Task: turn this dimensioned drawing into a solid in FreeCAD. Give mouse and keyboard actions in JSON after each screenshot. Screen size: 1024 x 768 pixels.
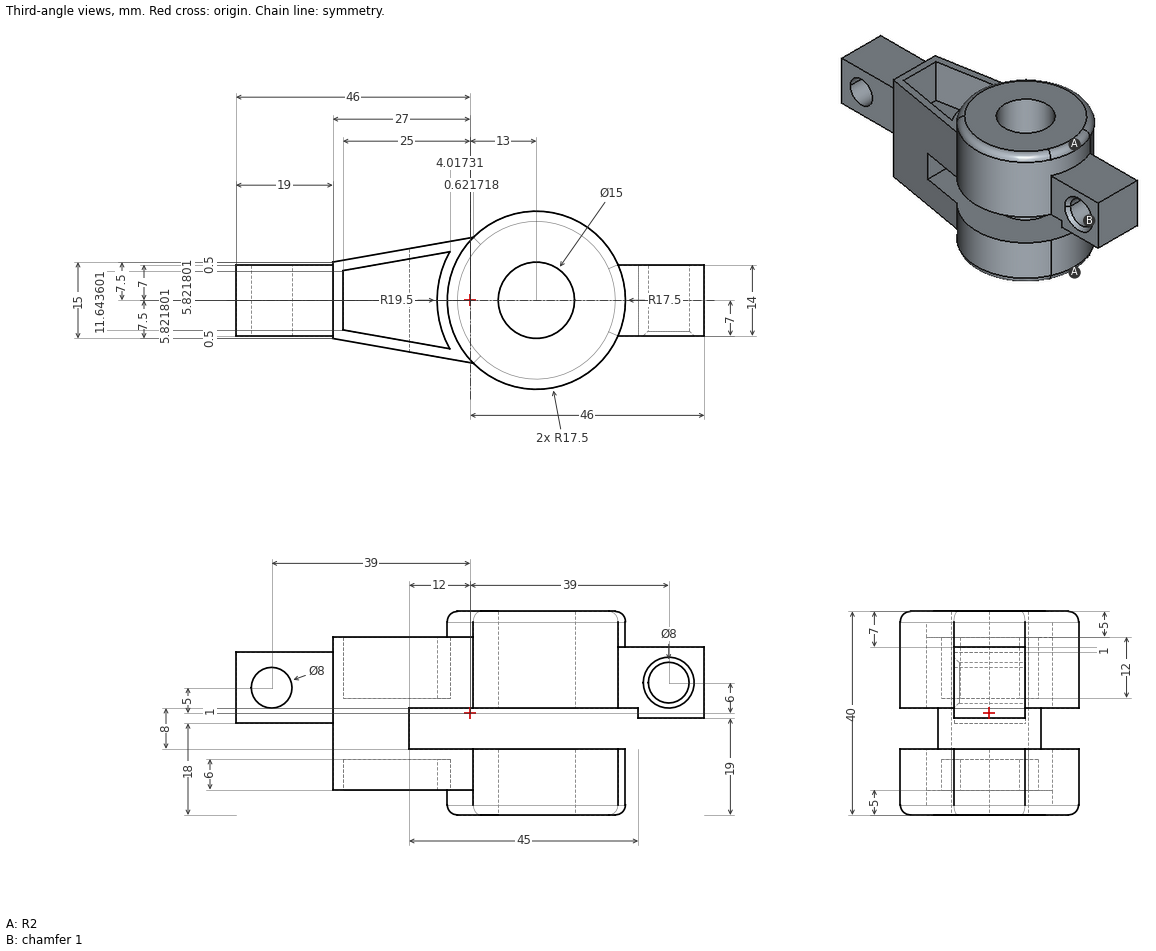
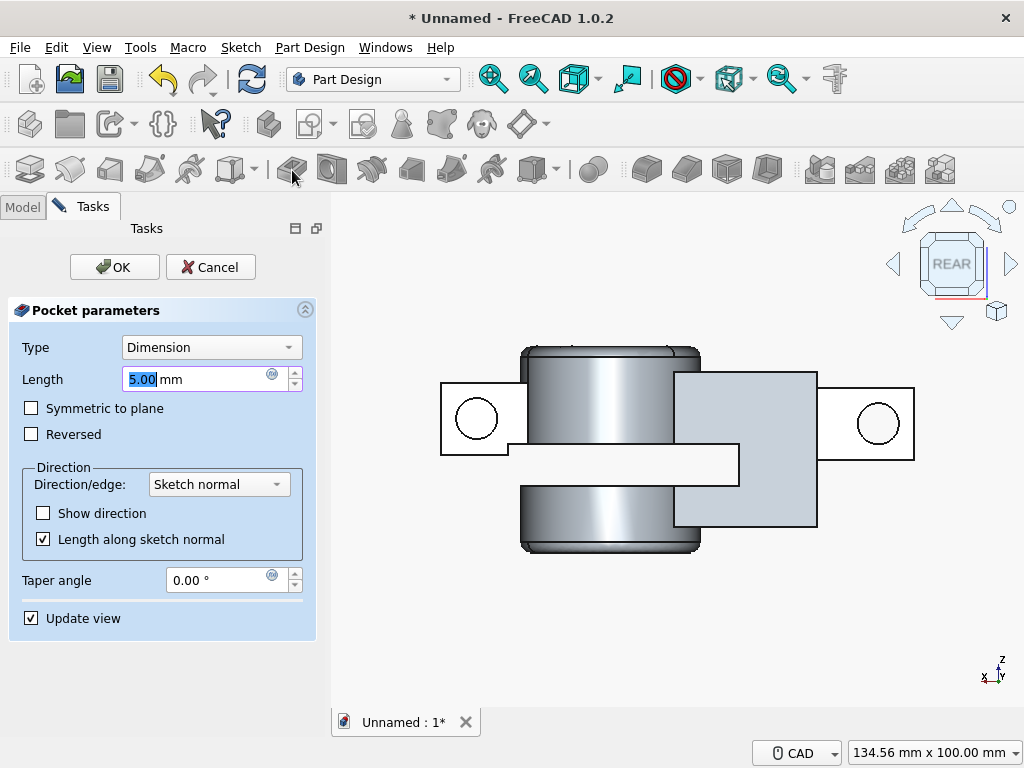
{"action": "left_click", "coordinate": [212, 348]}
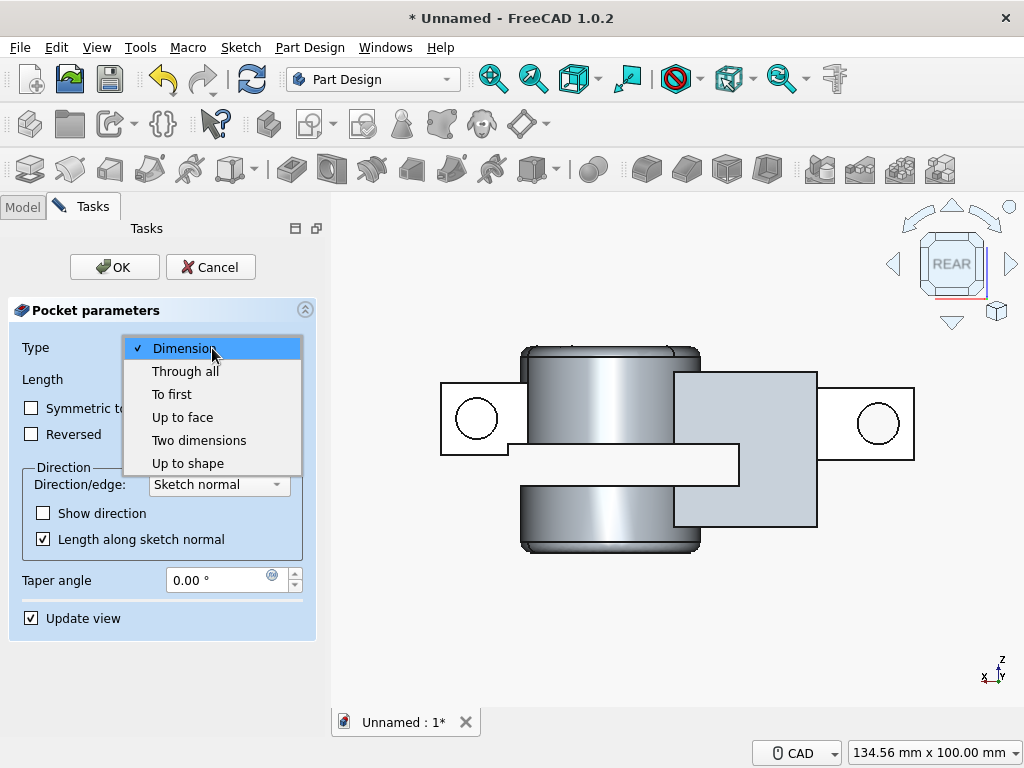
{"action": "left_click", "coordinate": [212, 394]}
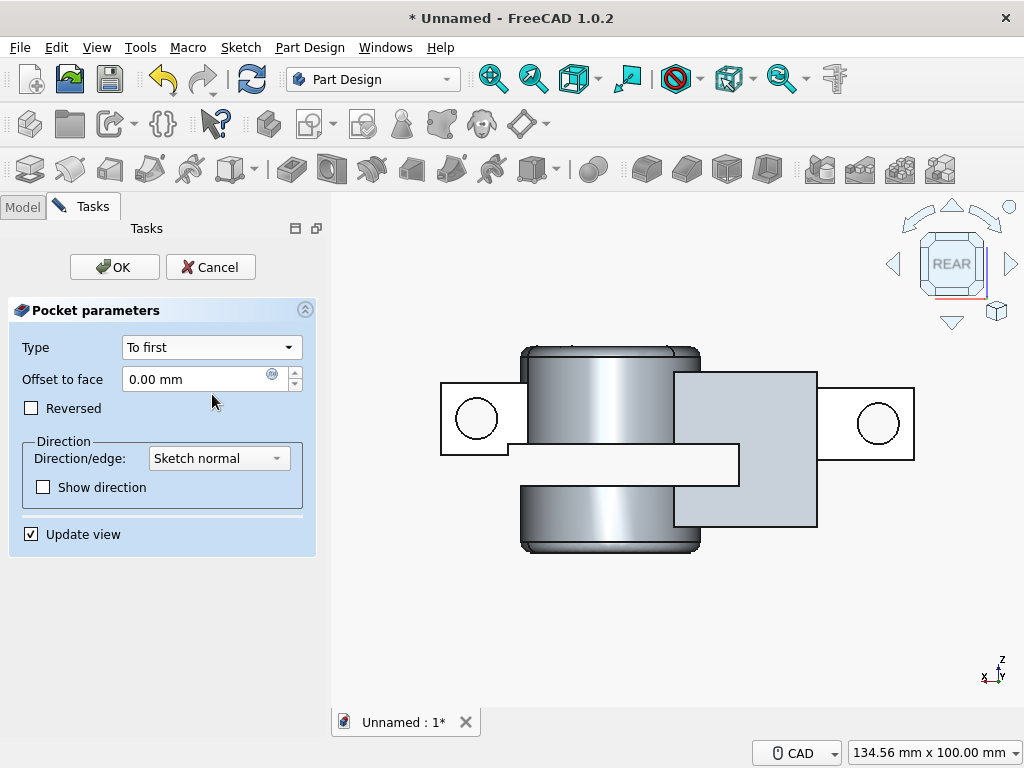
{"action": "left_click", "coordinate": [115, 267]}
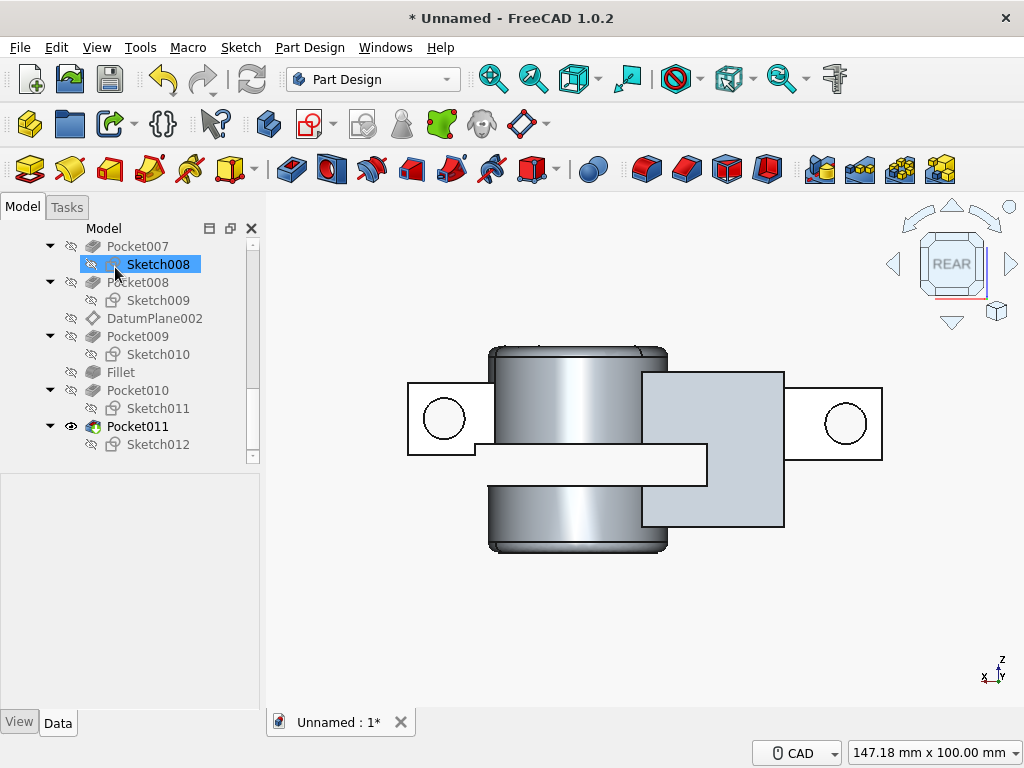
{"action": "key", "text": "0"}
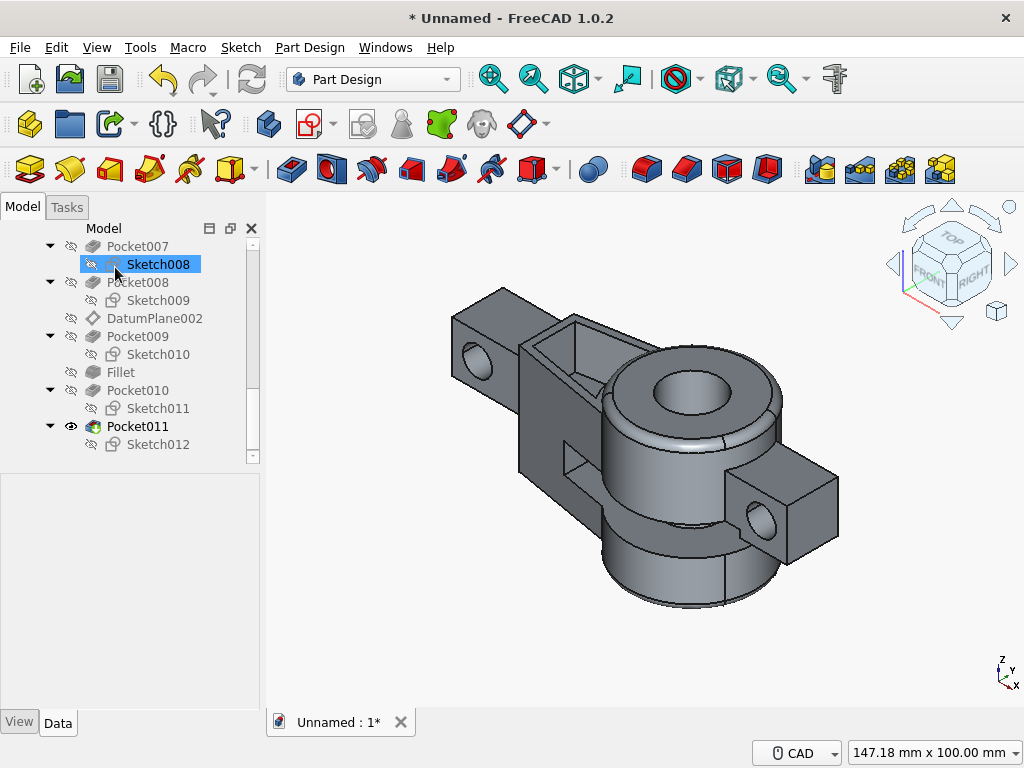
{"action": "left_click", "coordinate": [773, 537]}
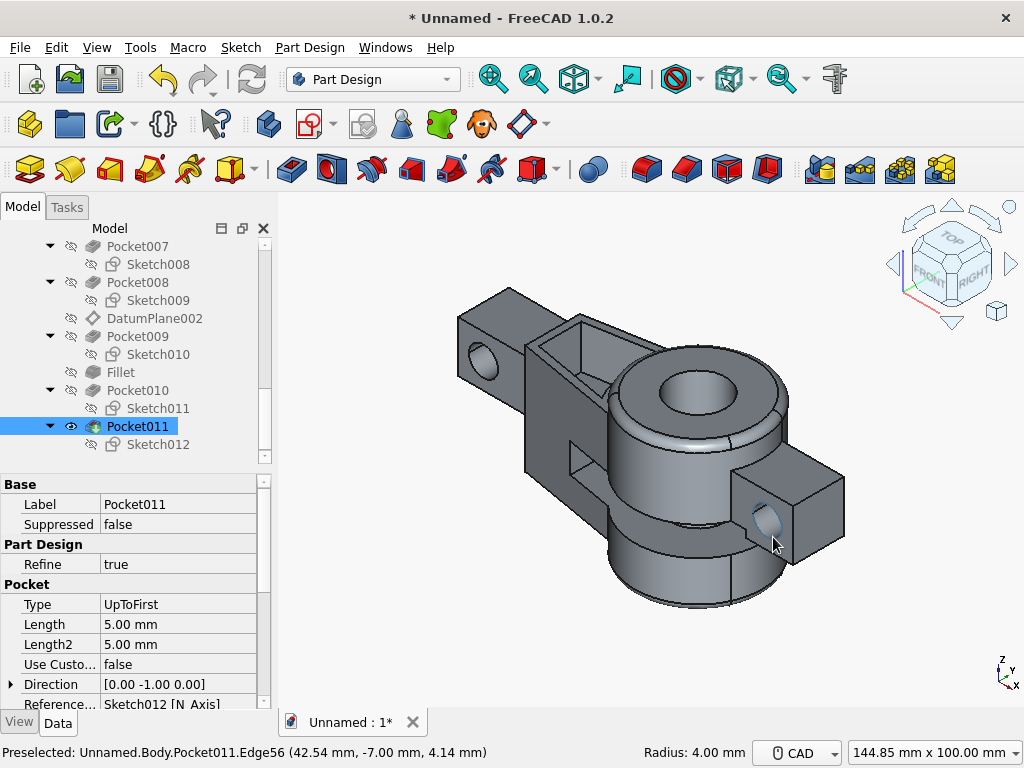
{"action": "left_click", "coordinate": [688, 170]}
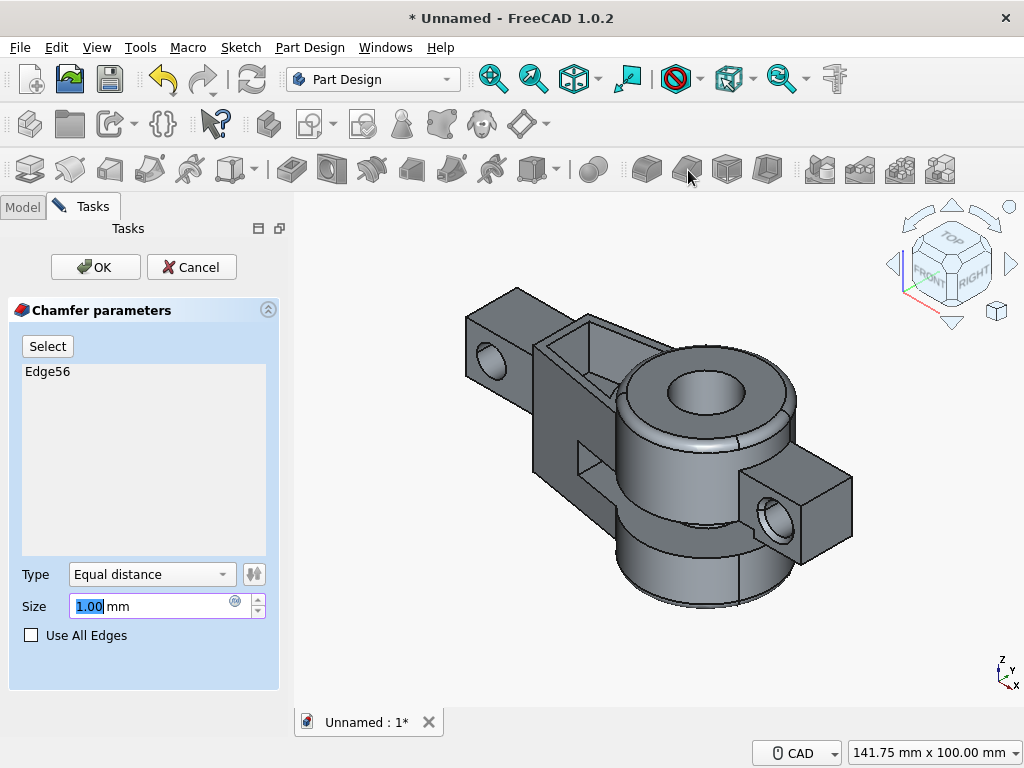
{"action": "type", "text": "1"}
{"action": "key", "text": "Tab"}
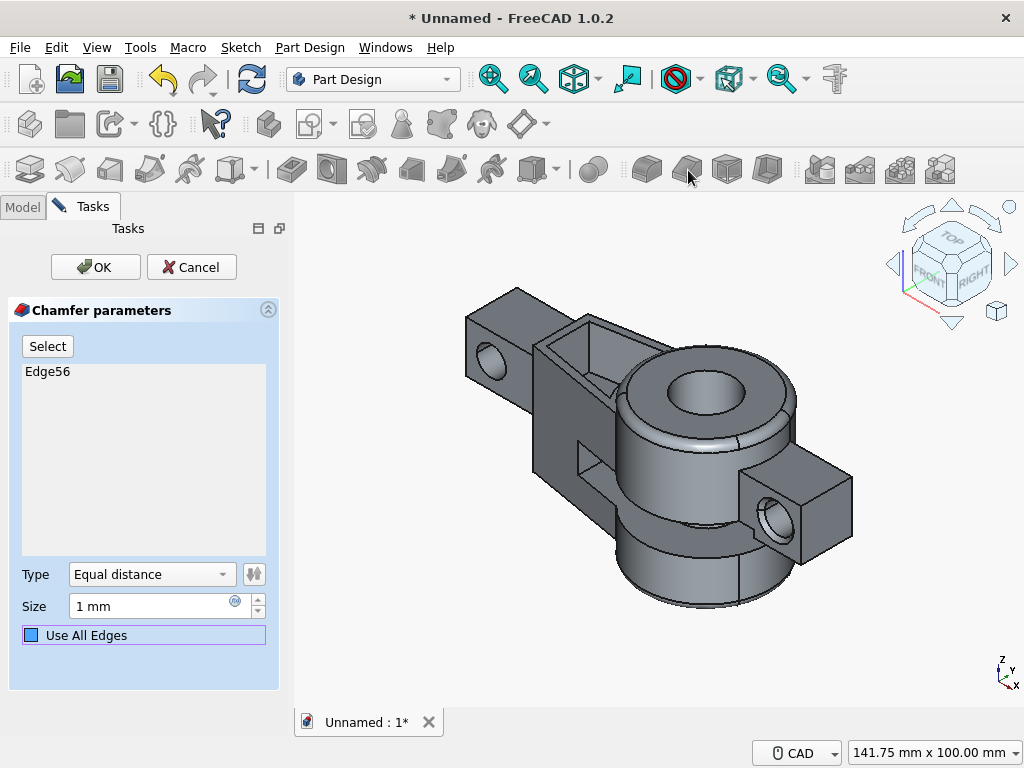
{"action": "left_click", "coordinate": [96, 267]}